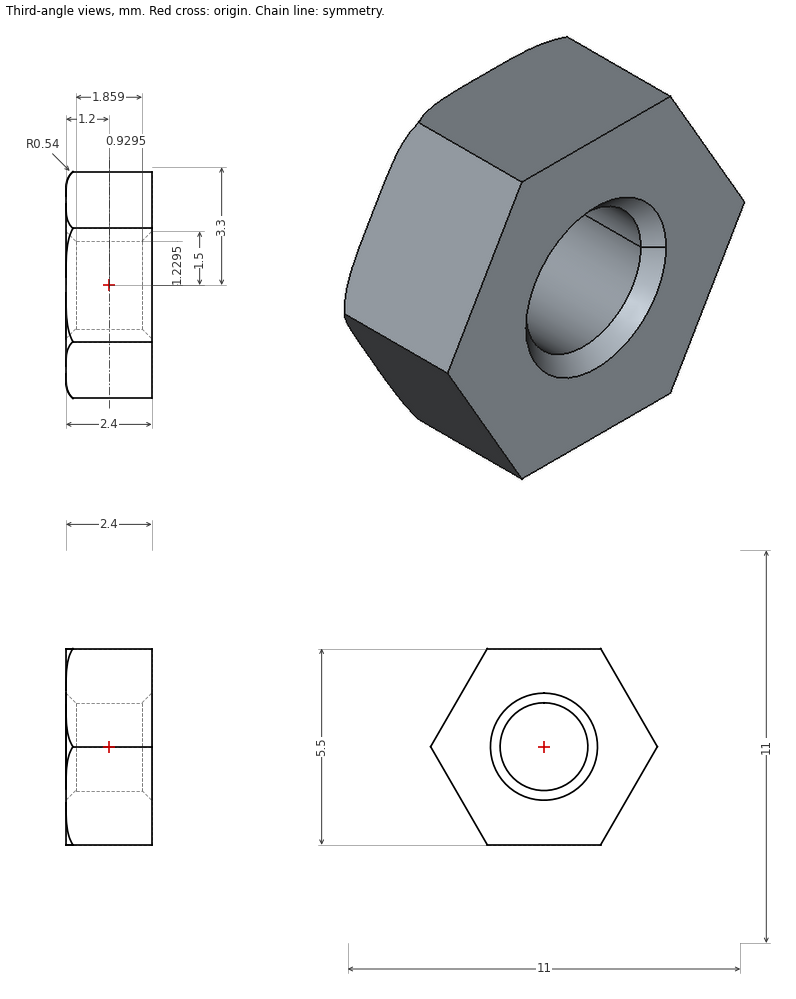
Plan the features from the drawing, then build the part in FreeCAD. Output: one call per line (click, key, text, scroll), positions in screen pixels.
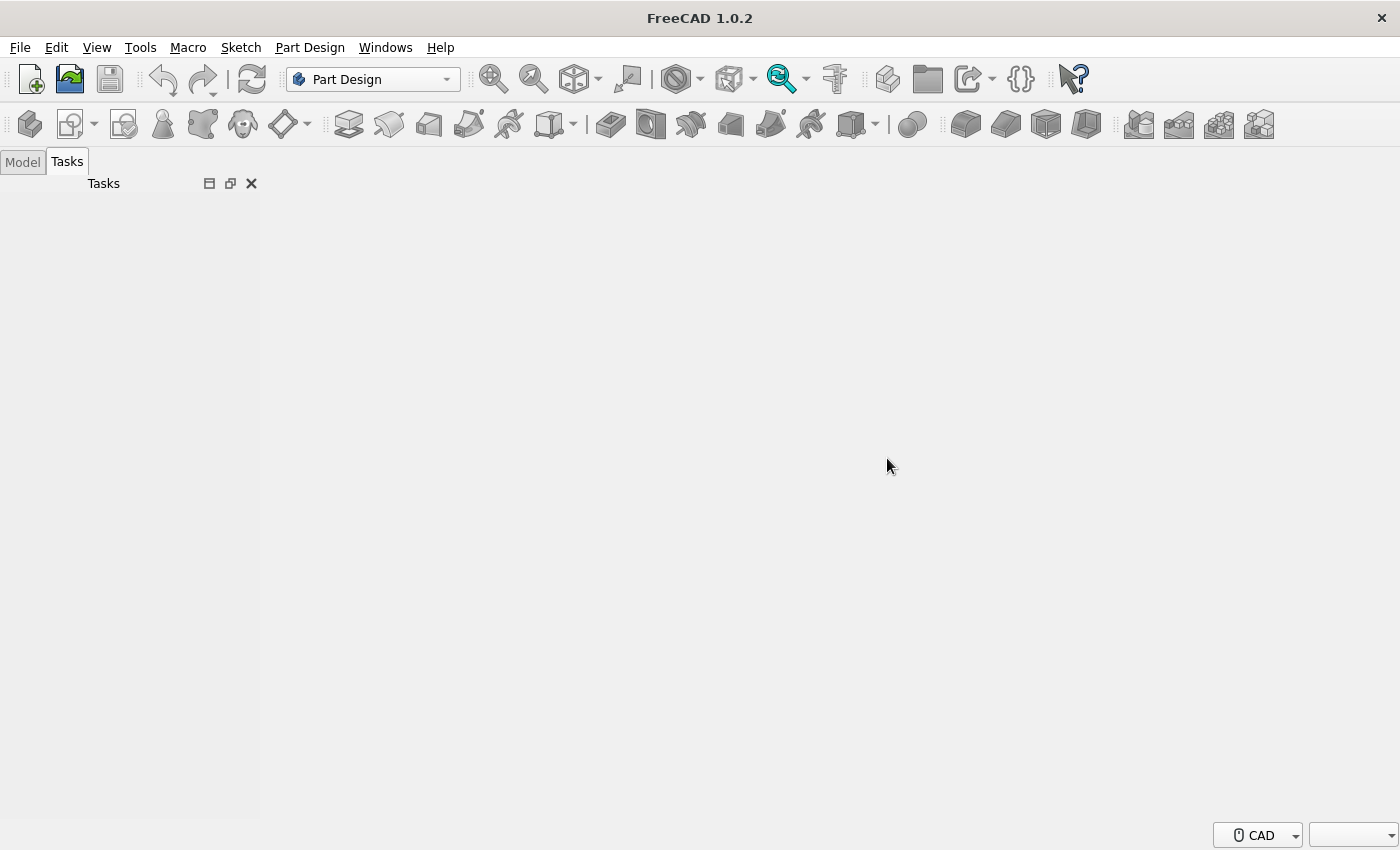
click(30, 80)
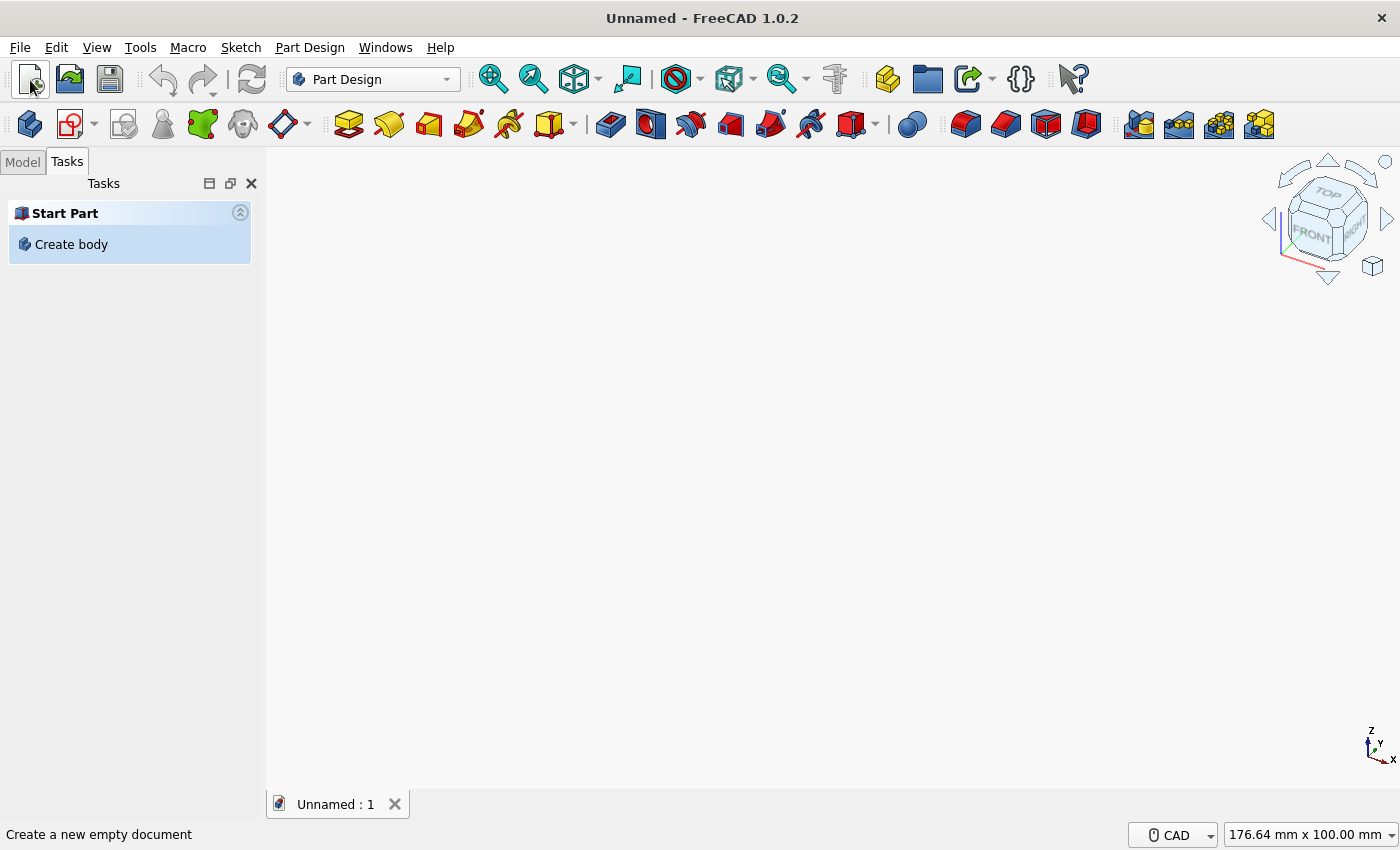
click(70, 124)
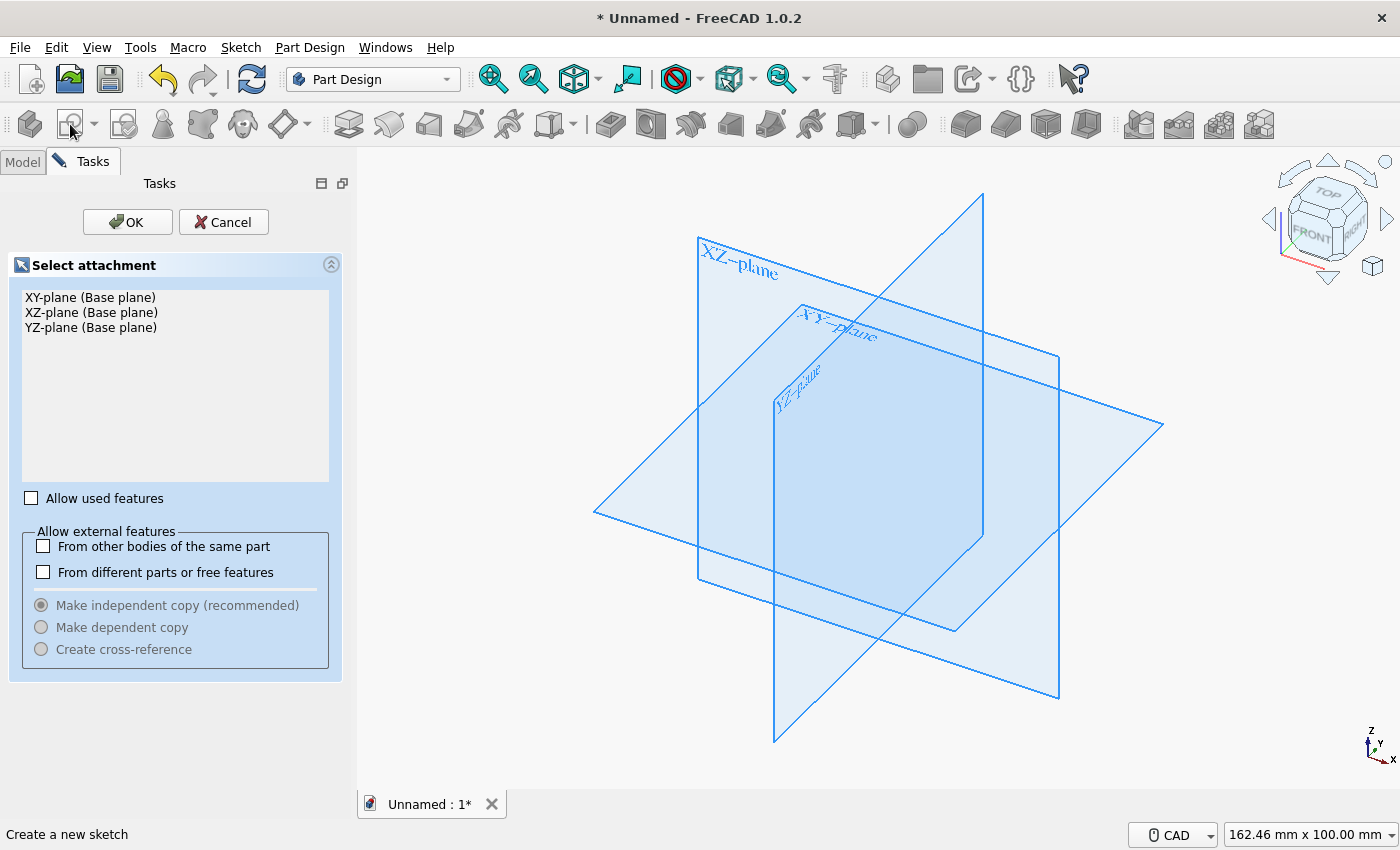
click(82, 298)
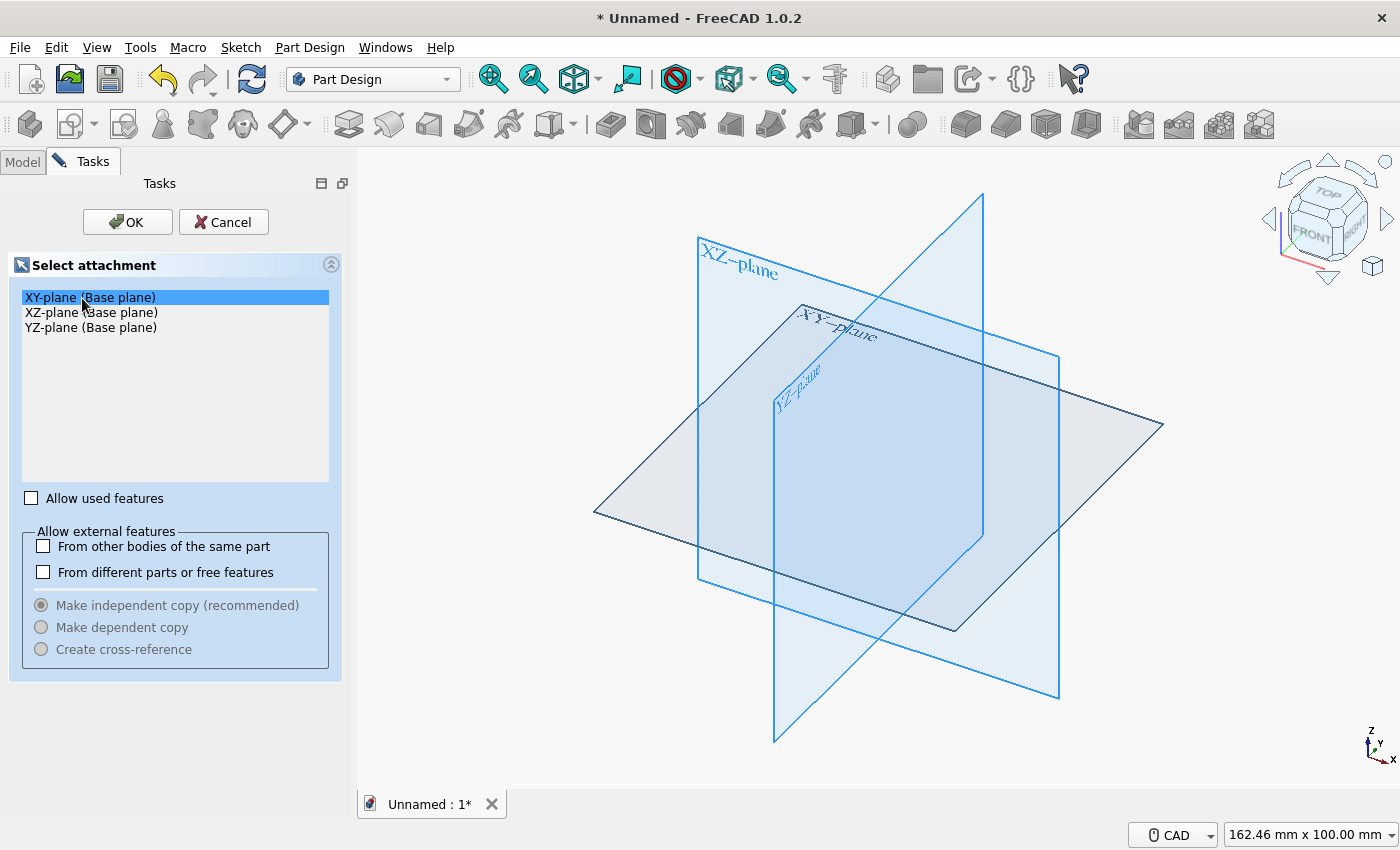
click(128, 222)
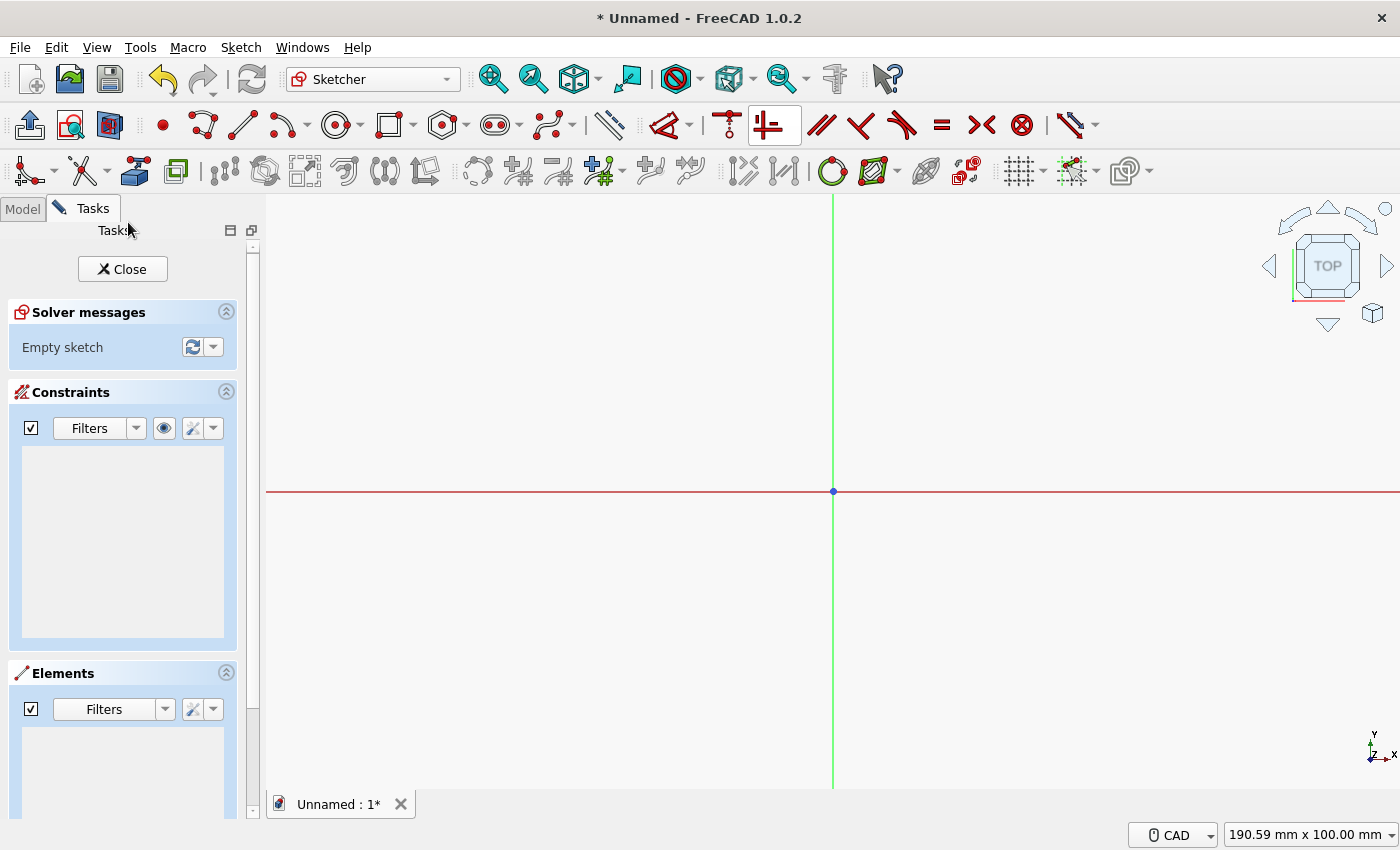
scroll(837, 481, up, 15)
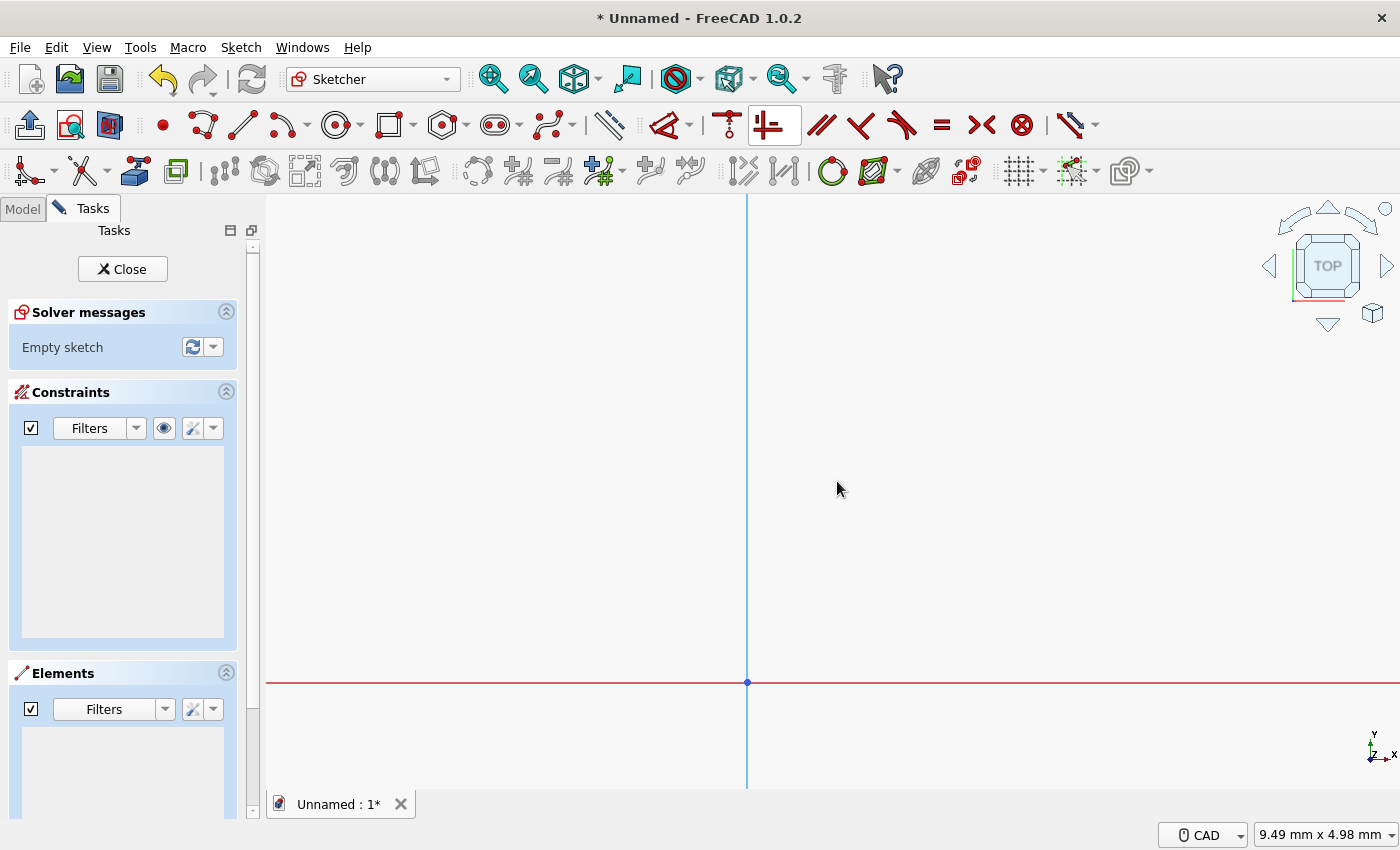
click(204, 126)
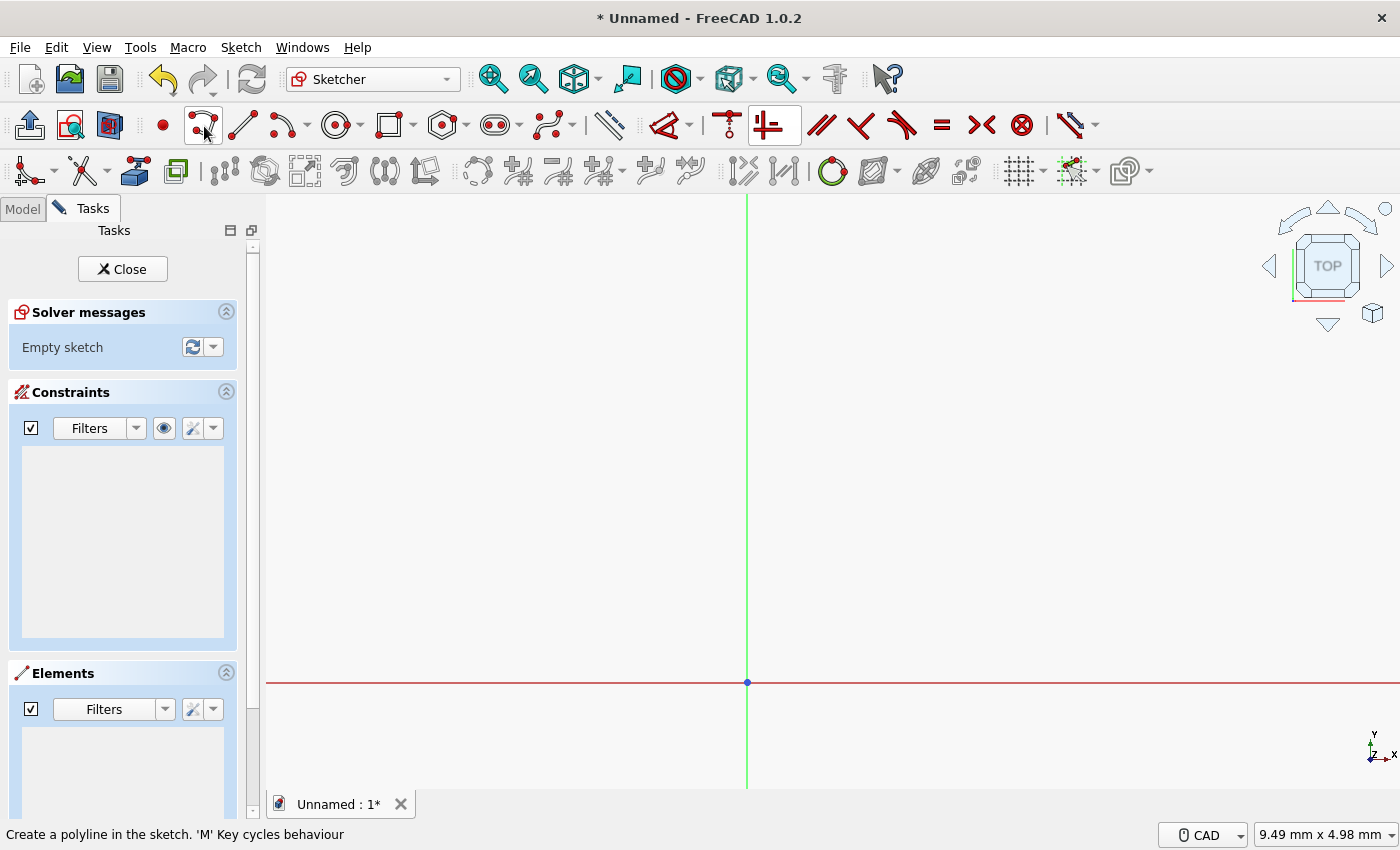
click(604, 353)
click(604, 683)
click(890, 674)
click(890, 288)
click(668, 288)
right_click(668, 288)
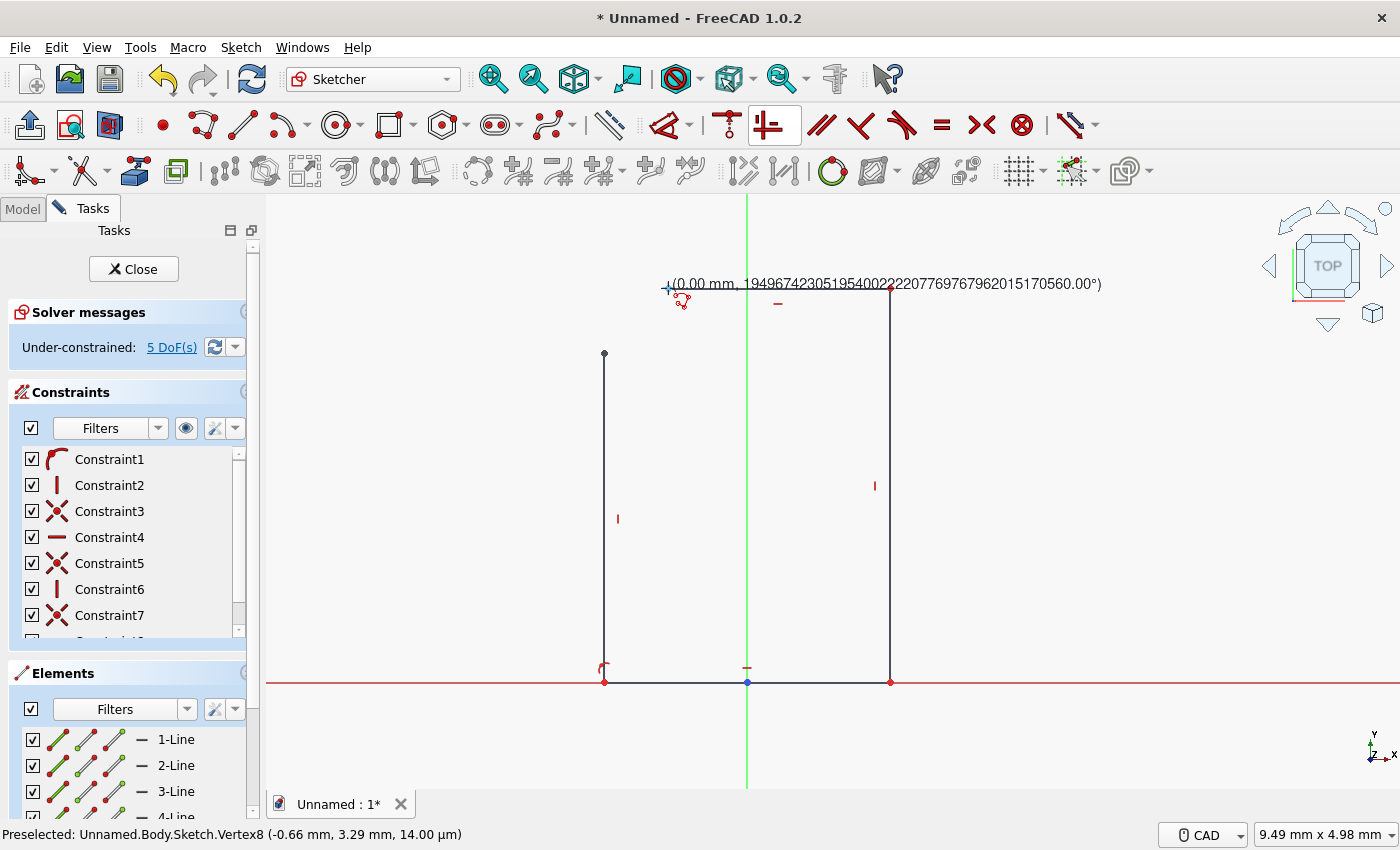
key(g)
key(3)
key(a)